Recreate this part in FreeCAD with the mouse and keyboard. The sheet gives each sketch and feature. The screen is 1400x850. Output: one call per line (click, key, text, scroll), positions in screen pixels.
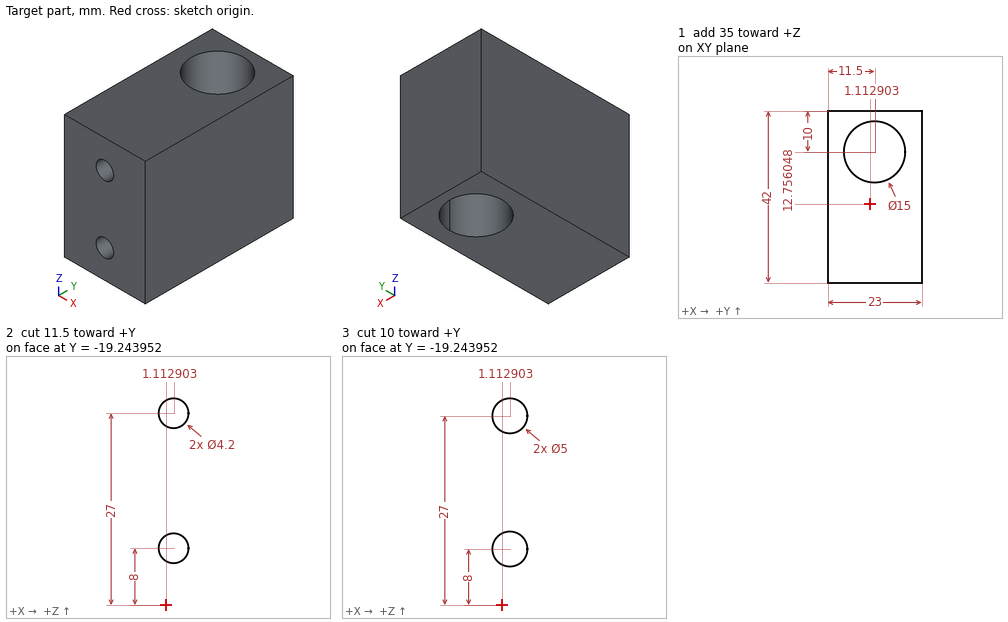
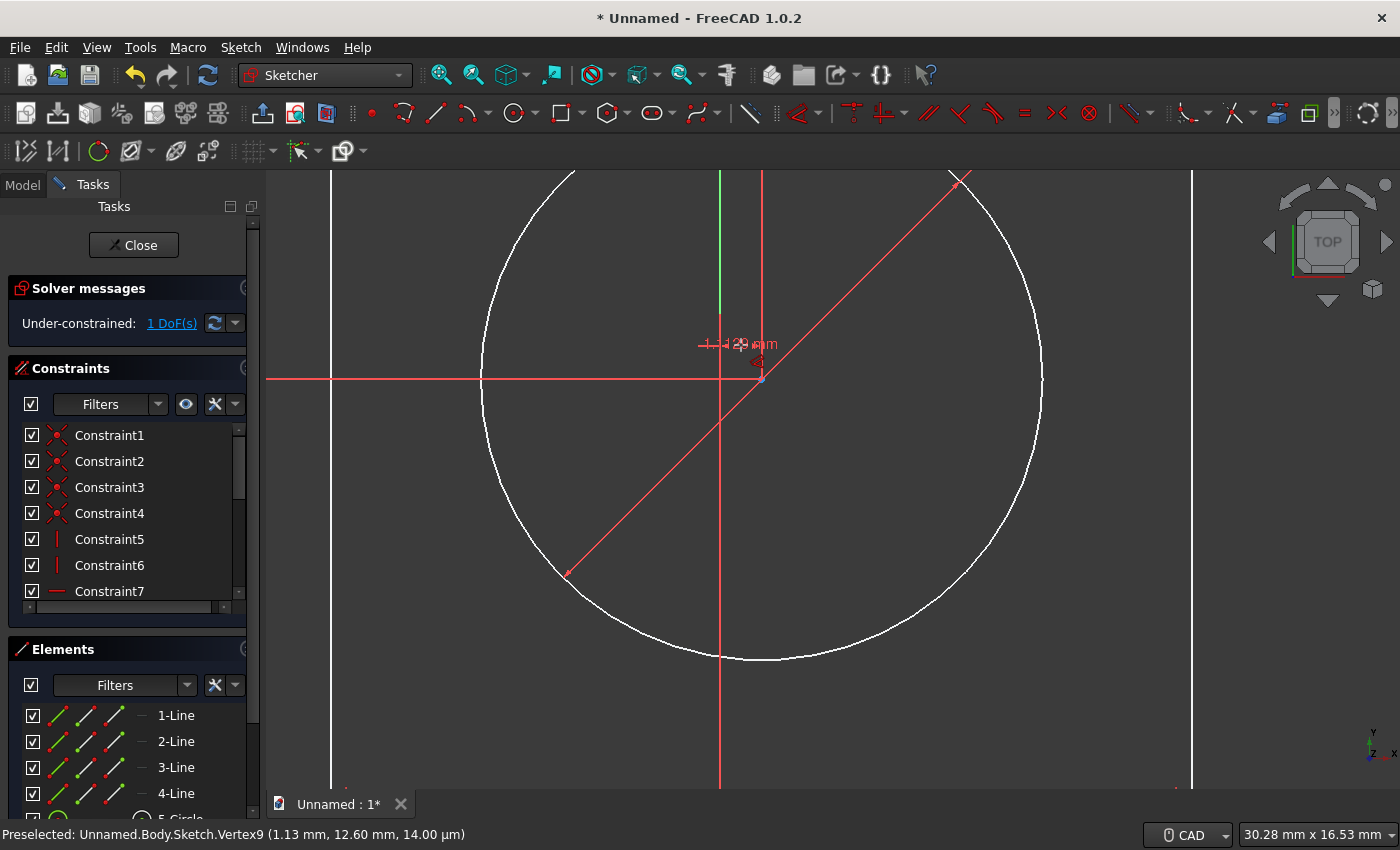
scroll(765, 379, down, 7)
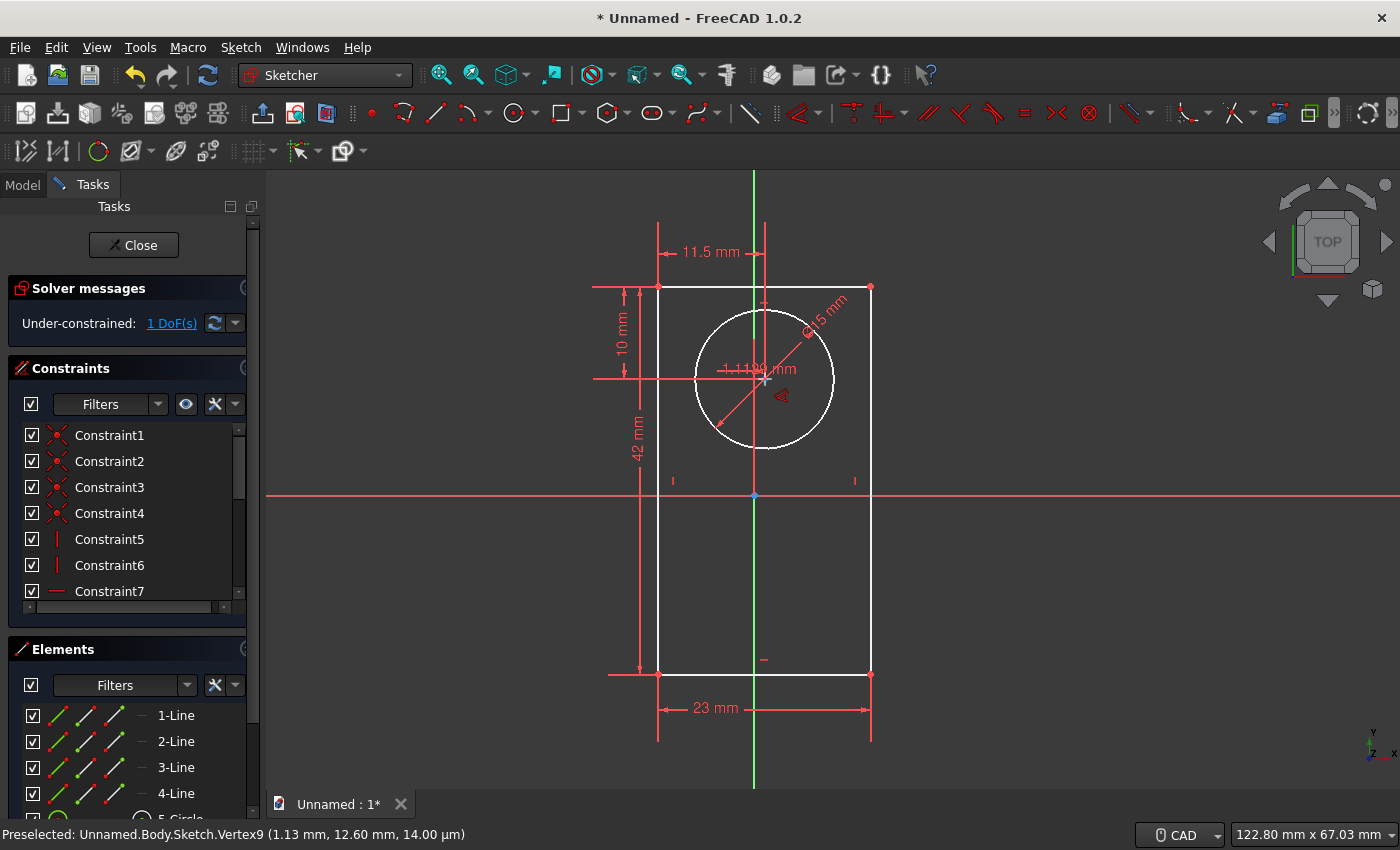
click(765, 379)
click(720, 411)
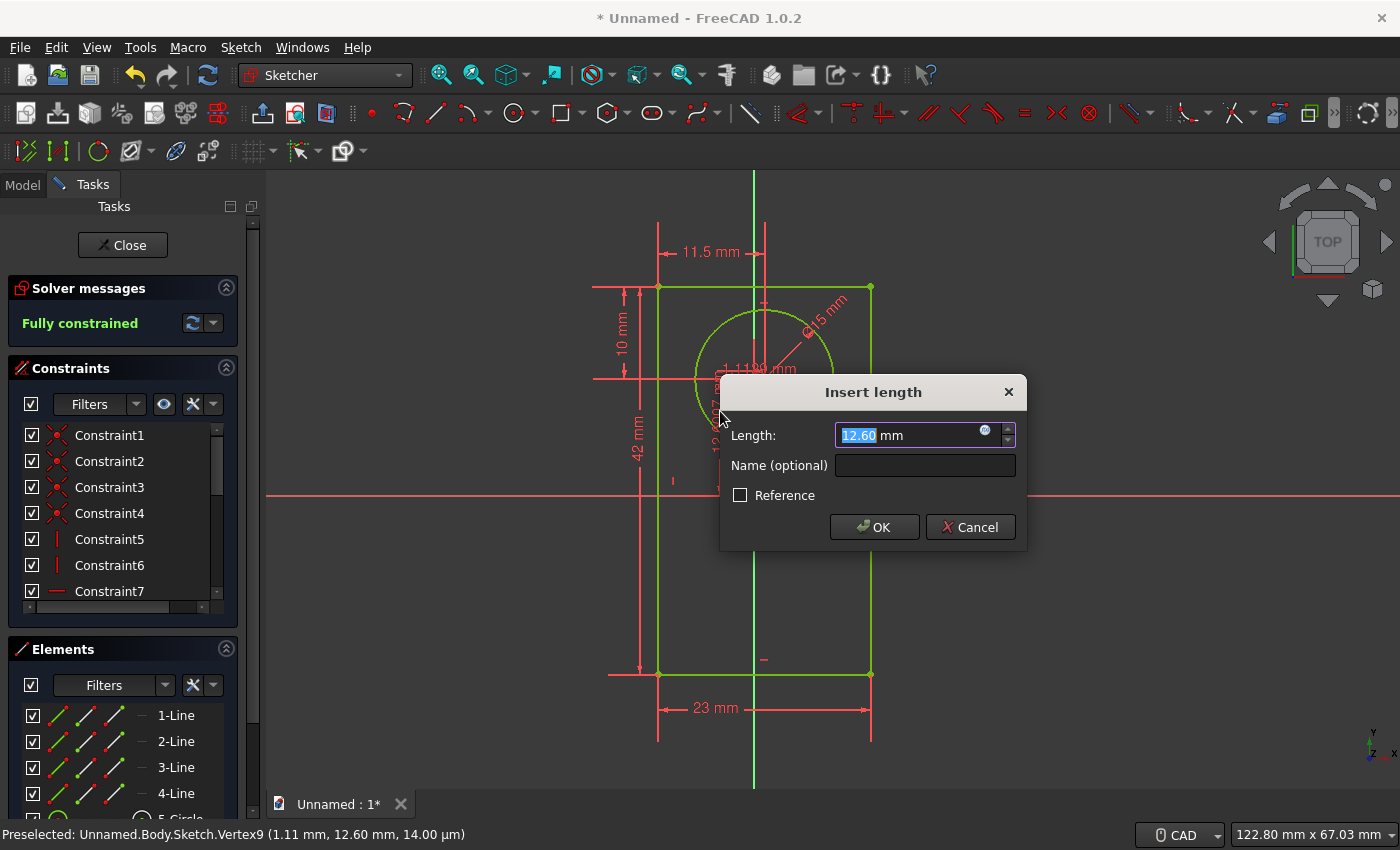
text(12.756048)
key(Return)
key(Escape)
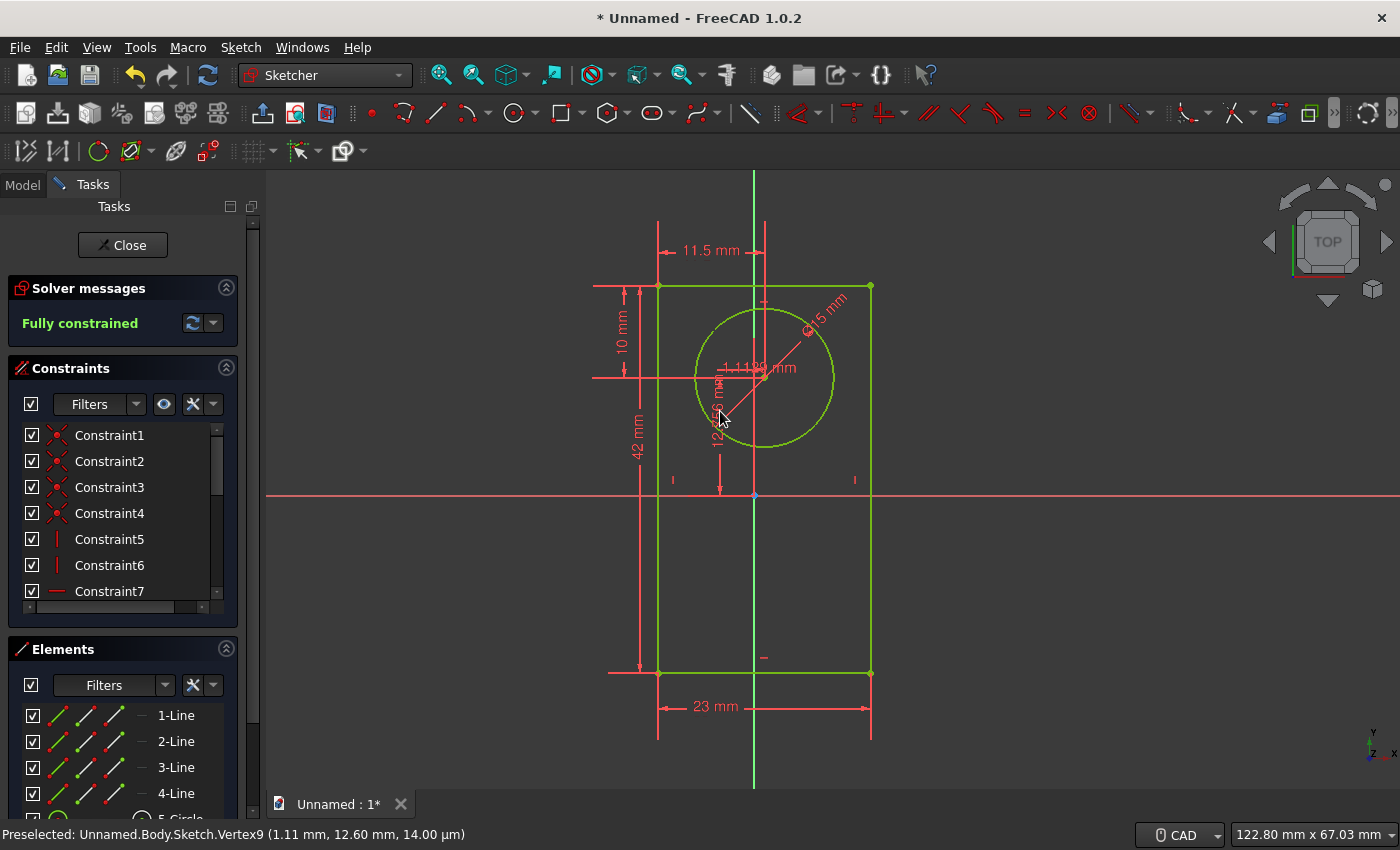
click(123, 245)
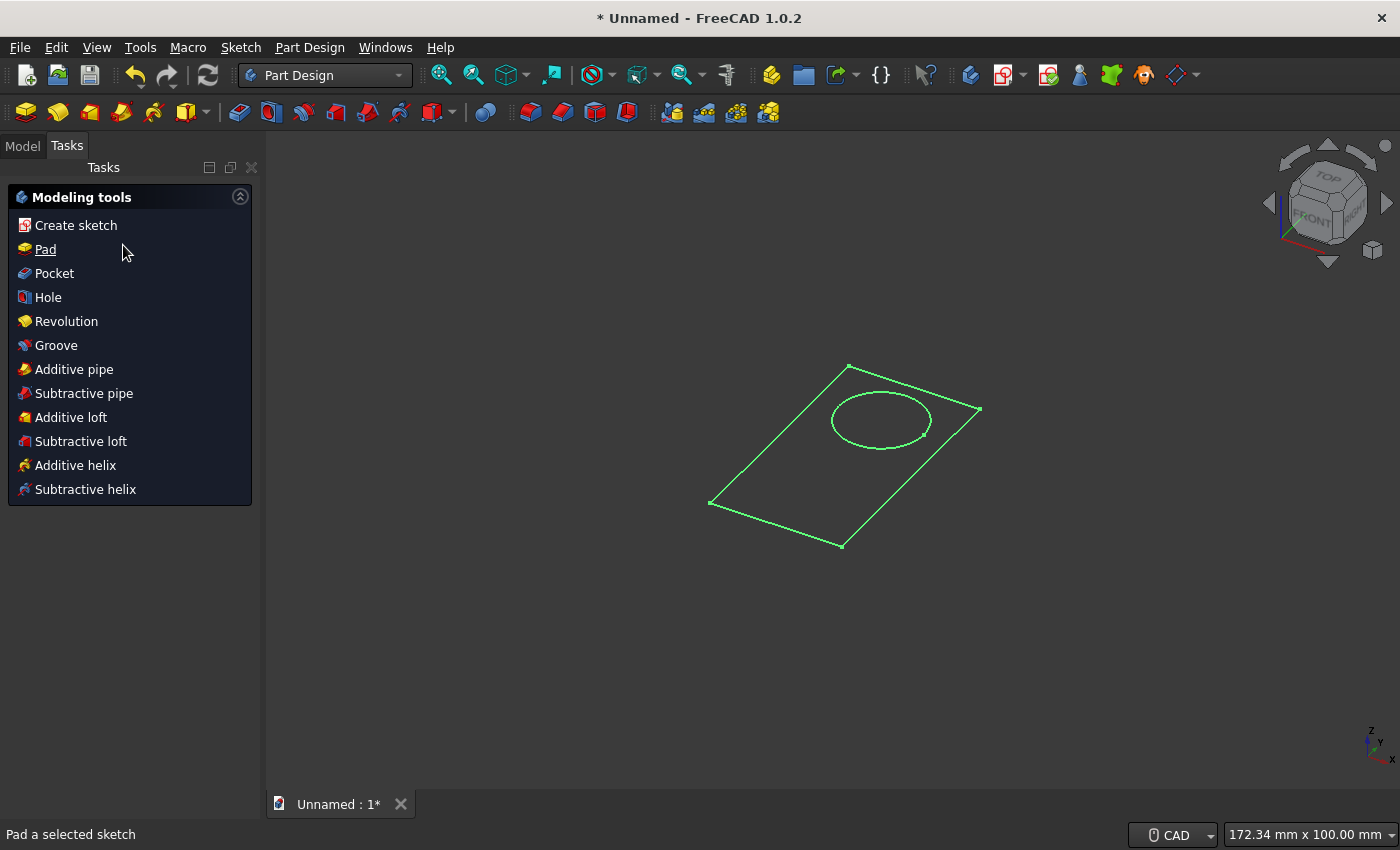
click(26, 112)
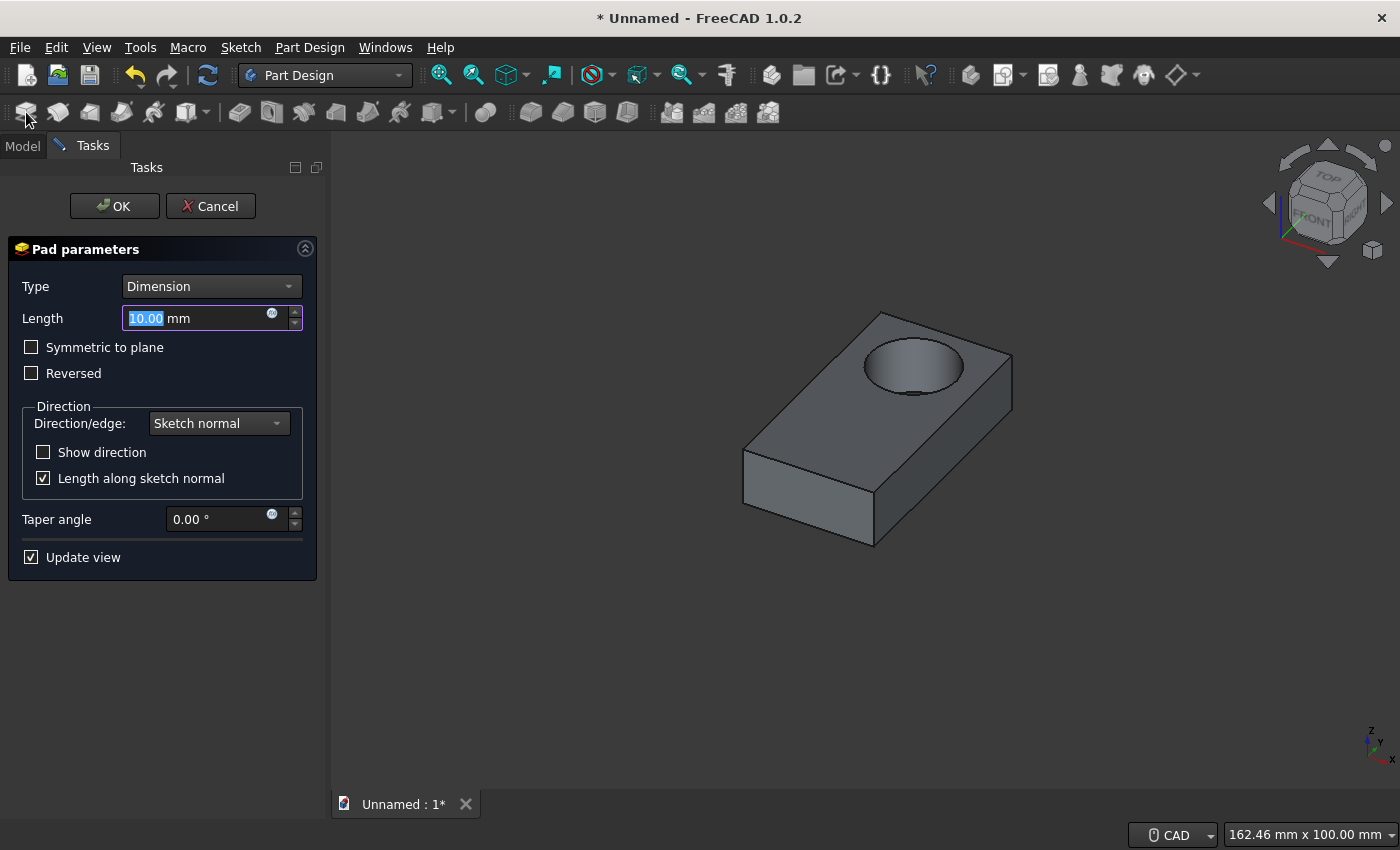
text(35)
key(Tab)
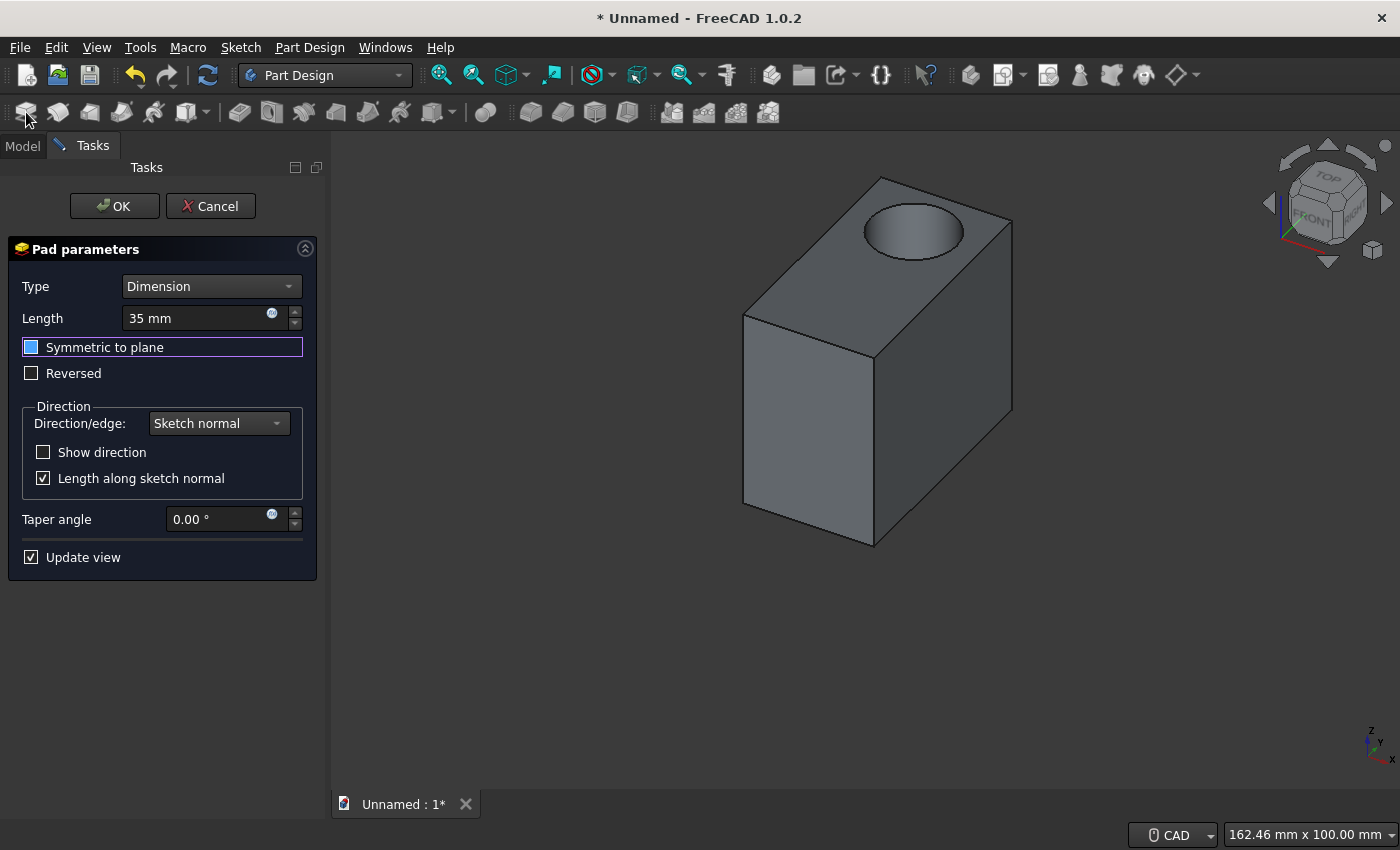
click(115, 206)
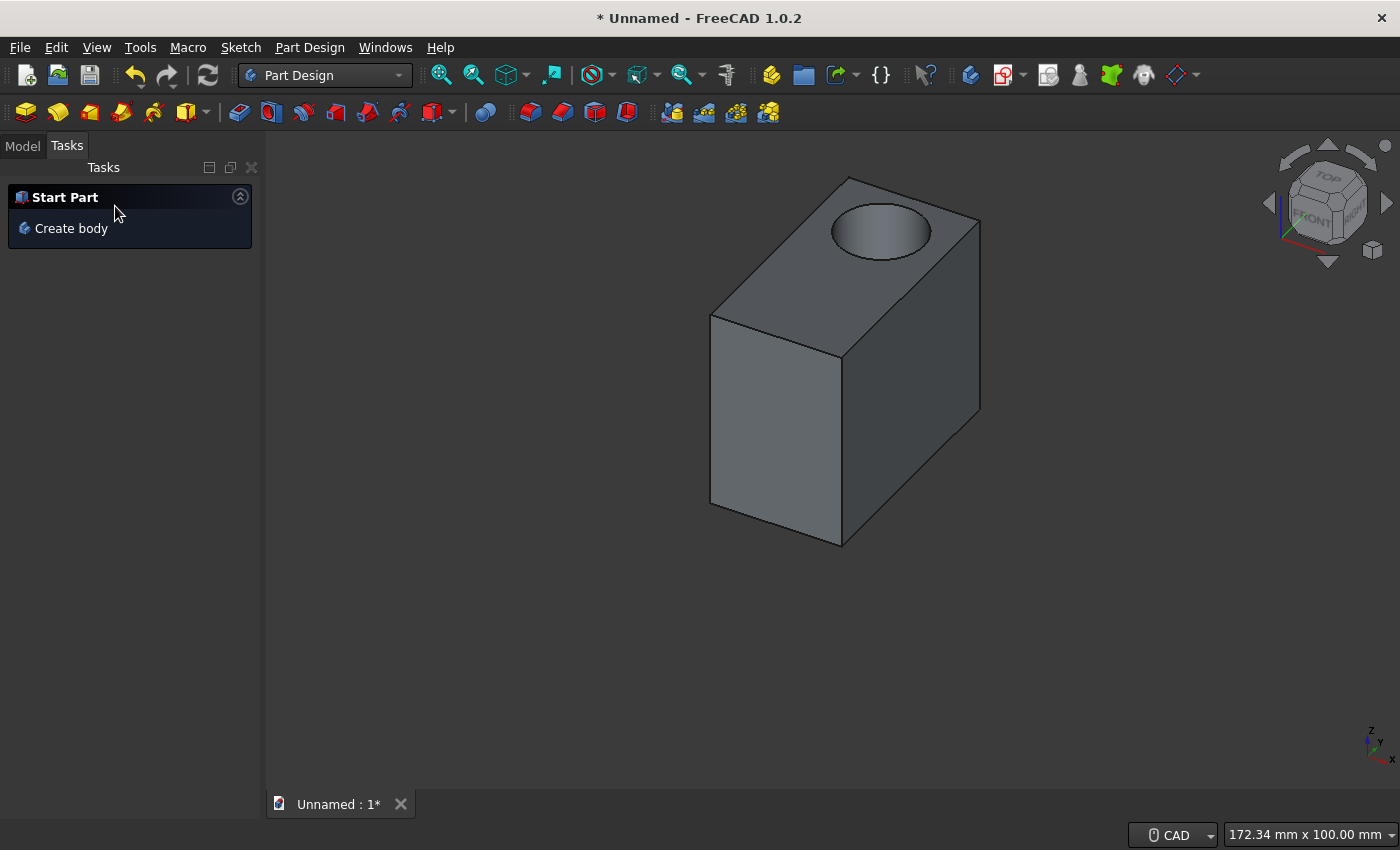
click(776, 403)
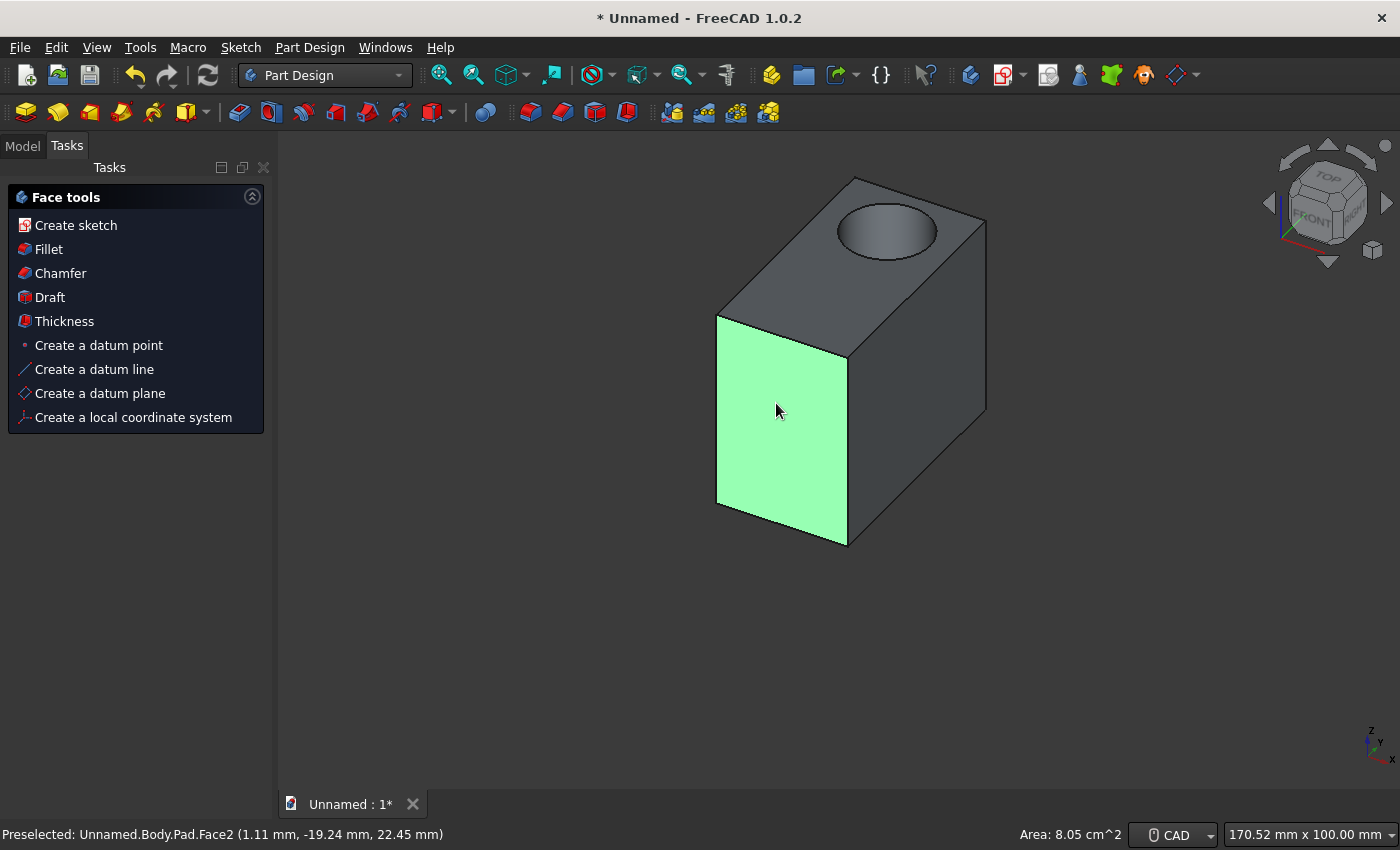
click(1004, 76)